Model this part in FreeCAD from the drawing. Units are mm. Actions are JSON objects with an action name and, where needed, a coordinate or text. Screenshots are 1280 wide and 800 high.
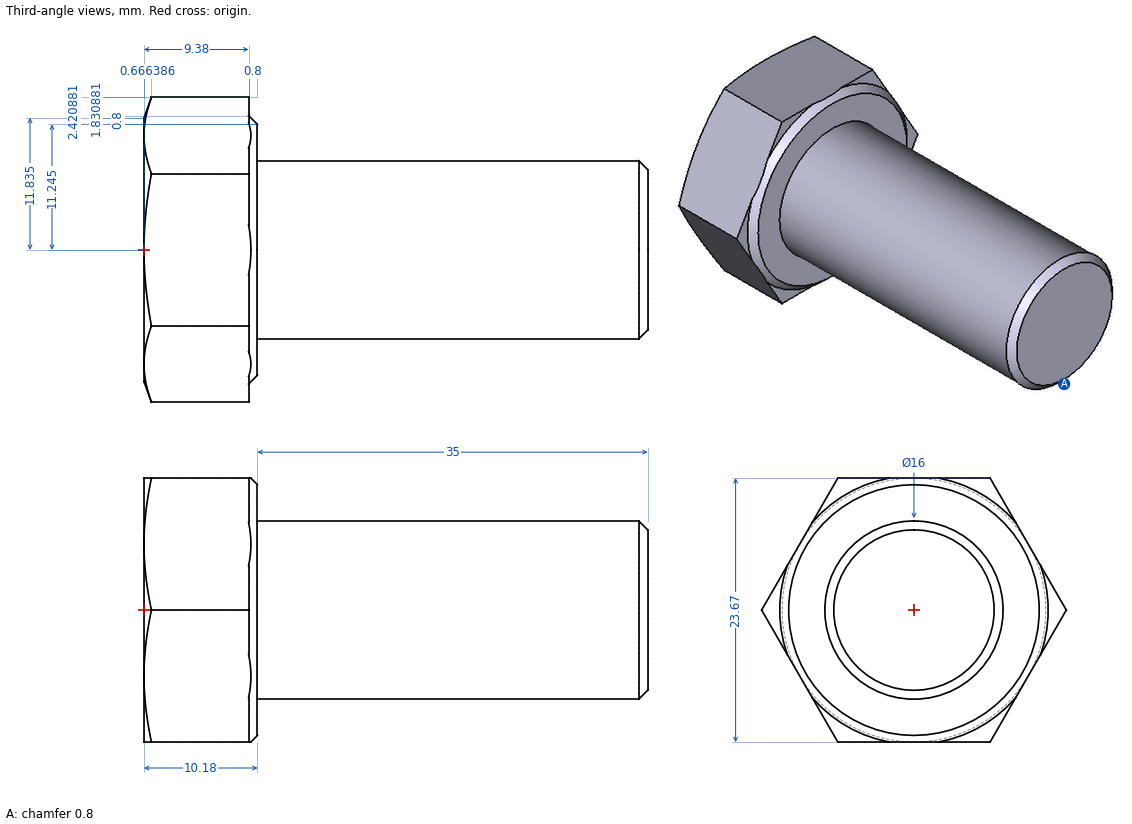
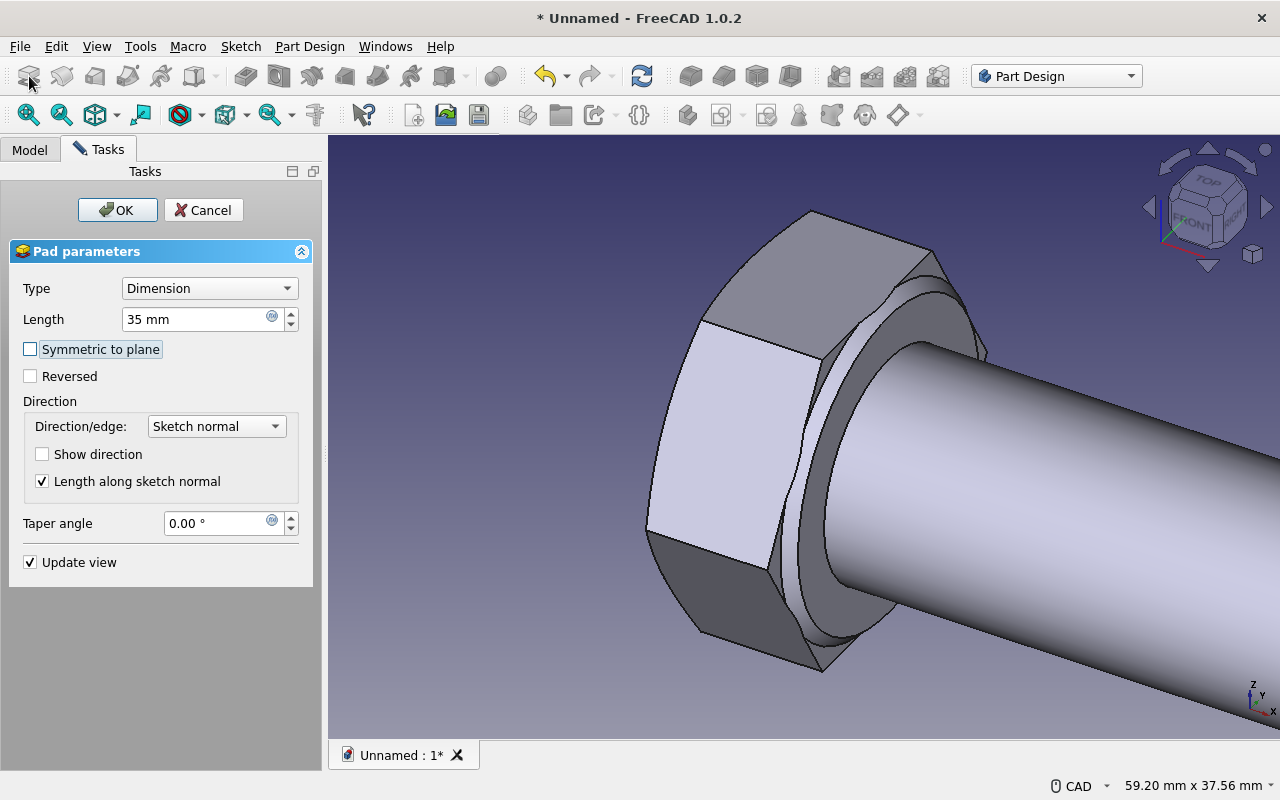
{"action": "left_click", "coordinate": [118, 210]}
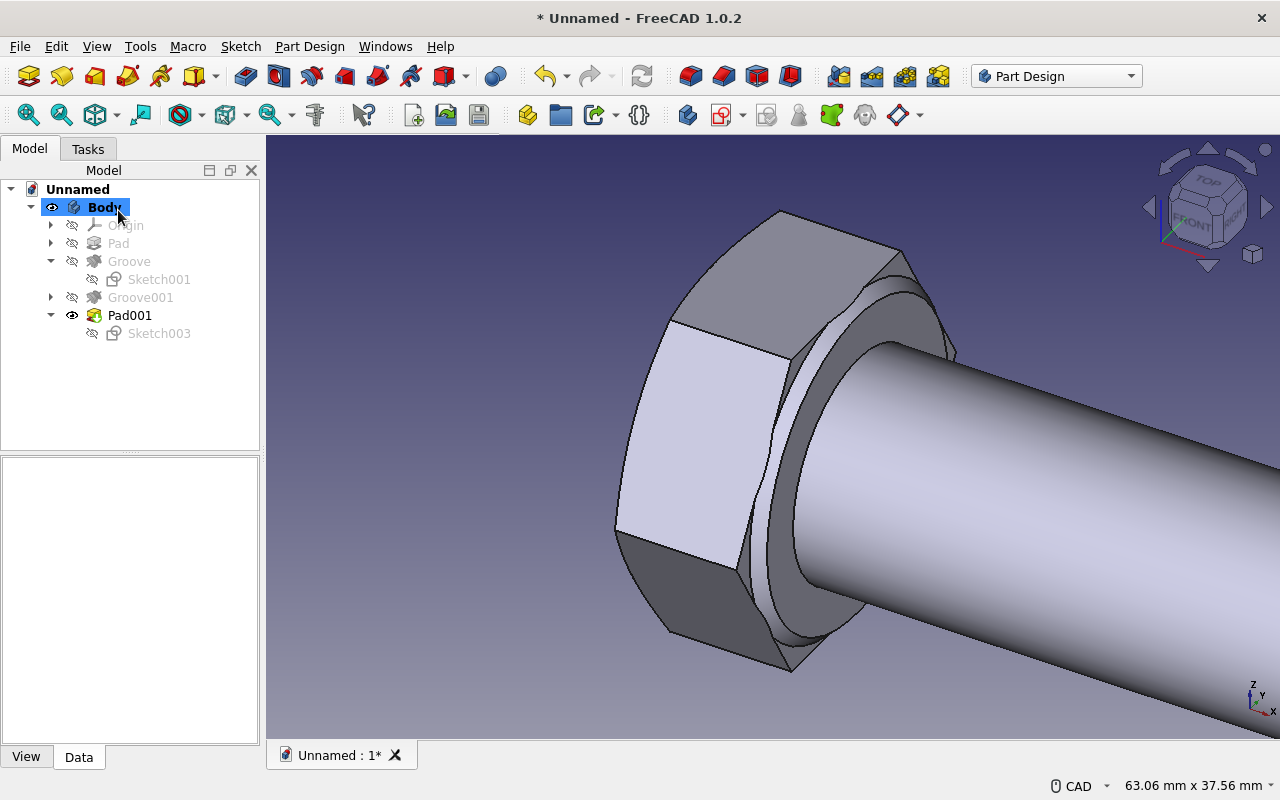
{"action": "left_click", "coordinate": [29, 116]}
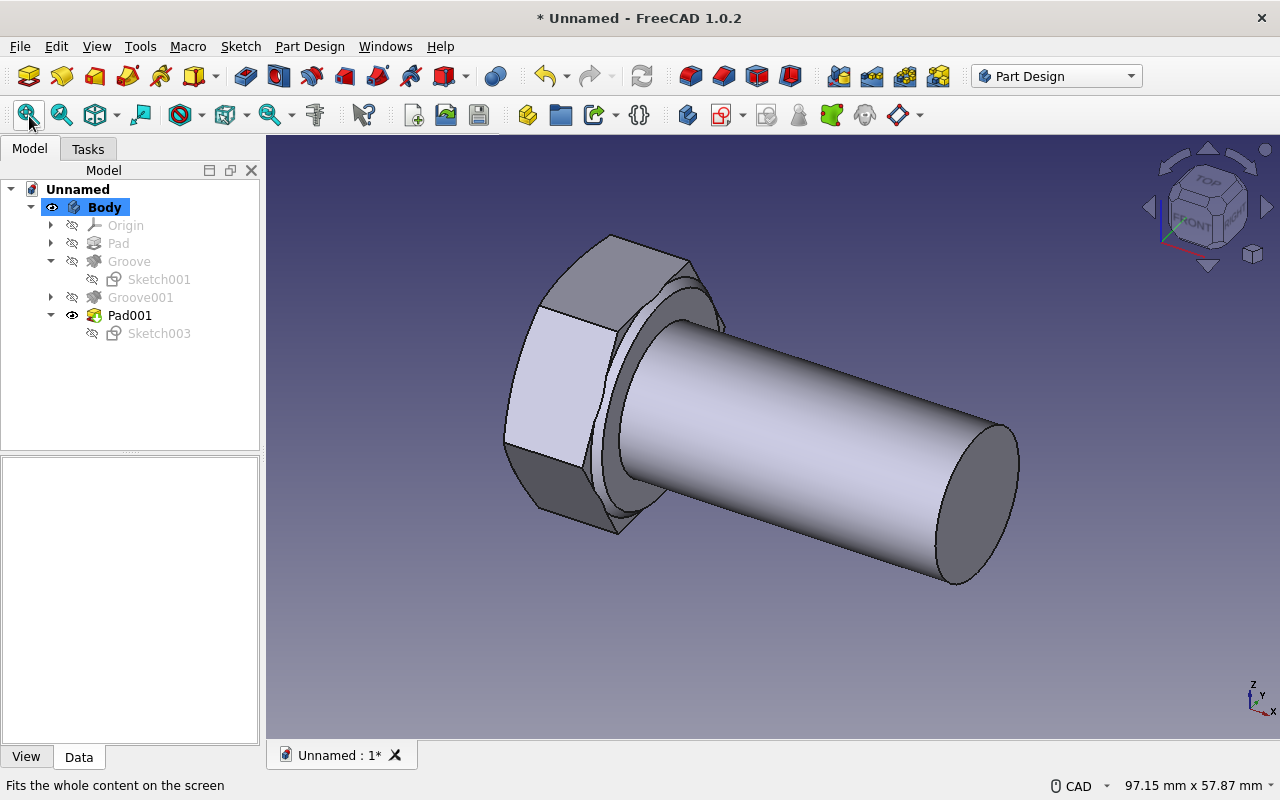
{"action": "left_click", "coordinate": [935, 545]}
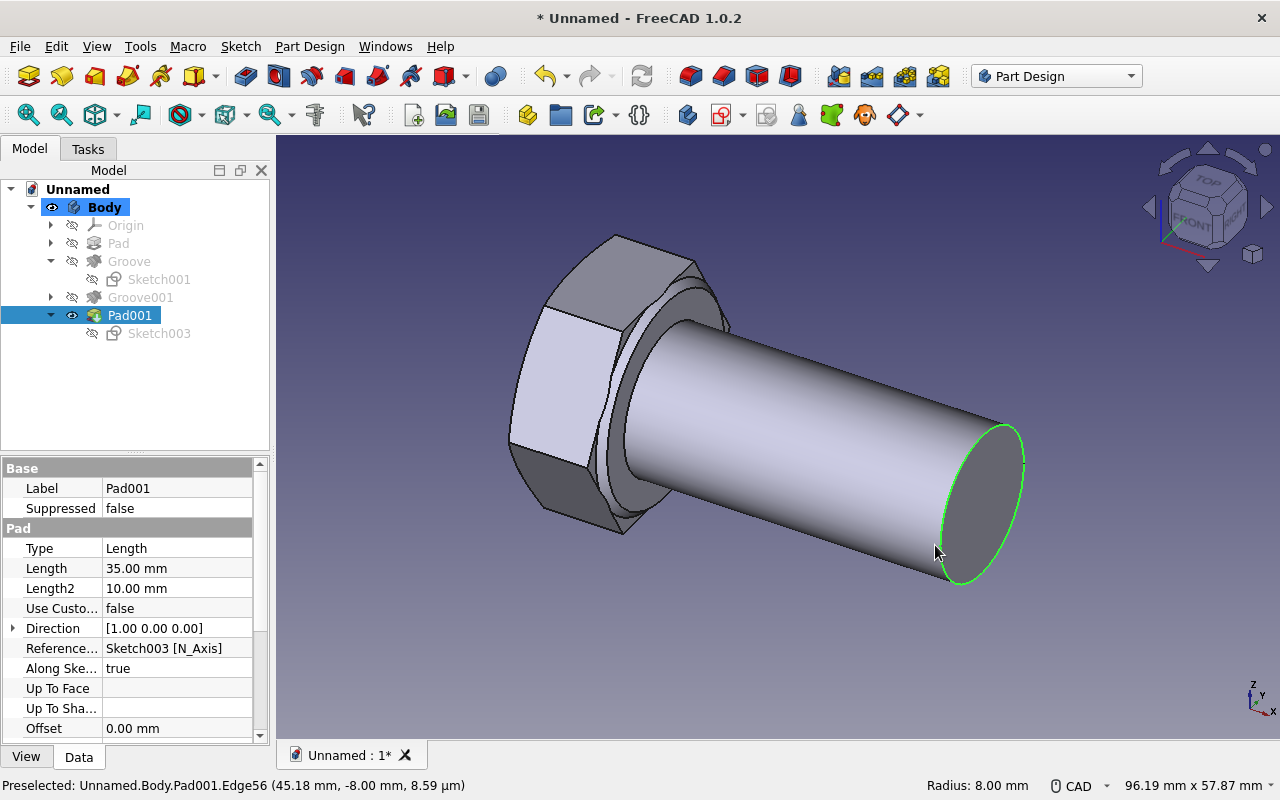
{"action": "left_click", "coordinate": [724, 76]}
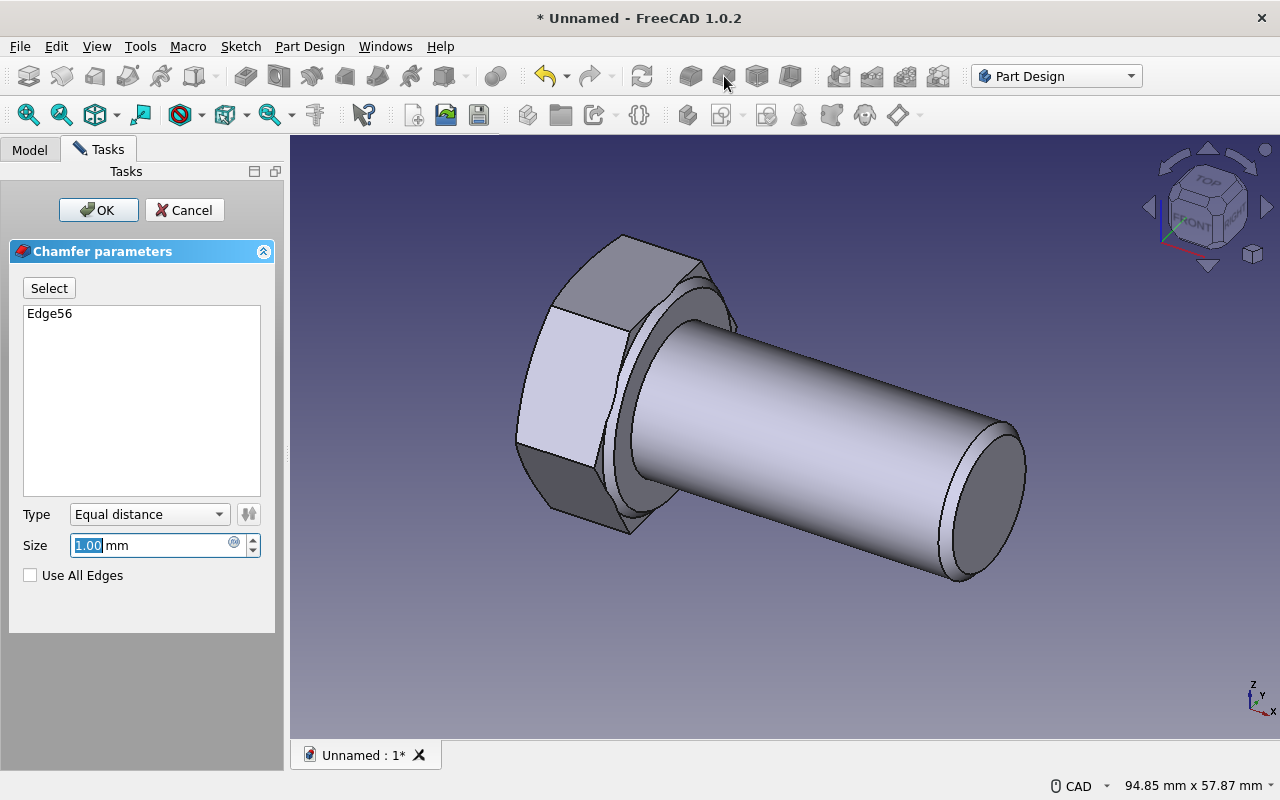
{"action": "type", "text": "0.8"}
{"action": "key", "text": "Tab"}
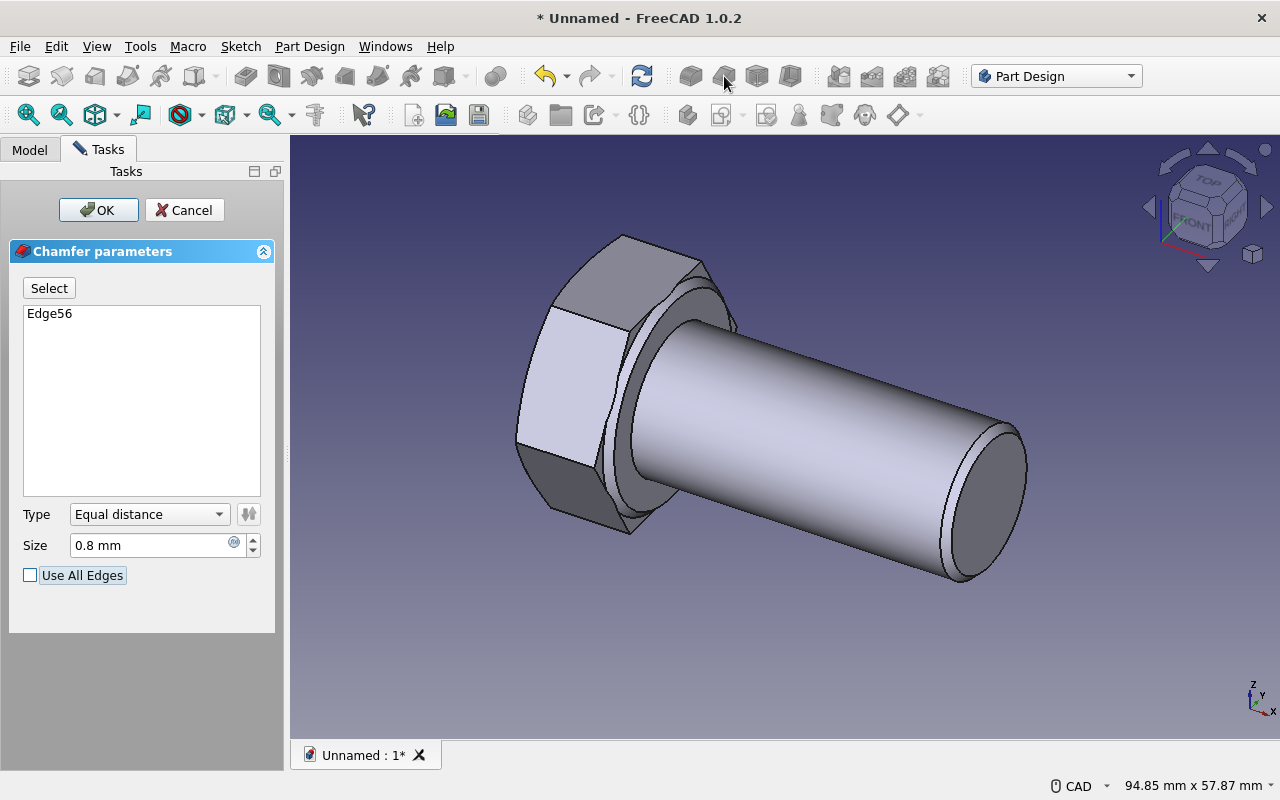
{"action": "left_click", "coordinate": [99, 210]}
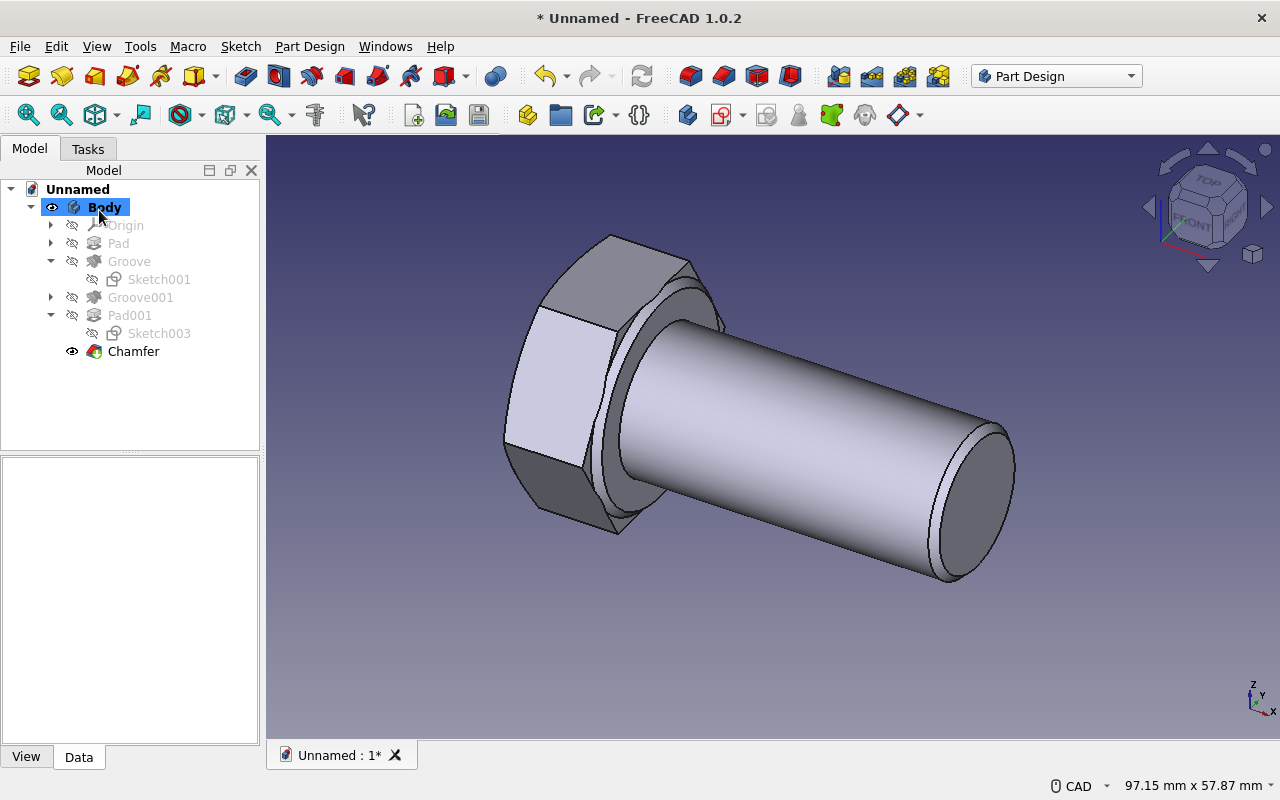
{"action": "key", "text": "0"}